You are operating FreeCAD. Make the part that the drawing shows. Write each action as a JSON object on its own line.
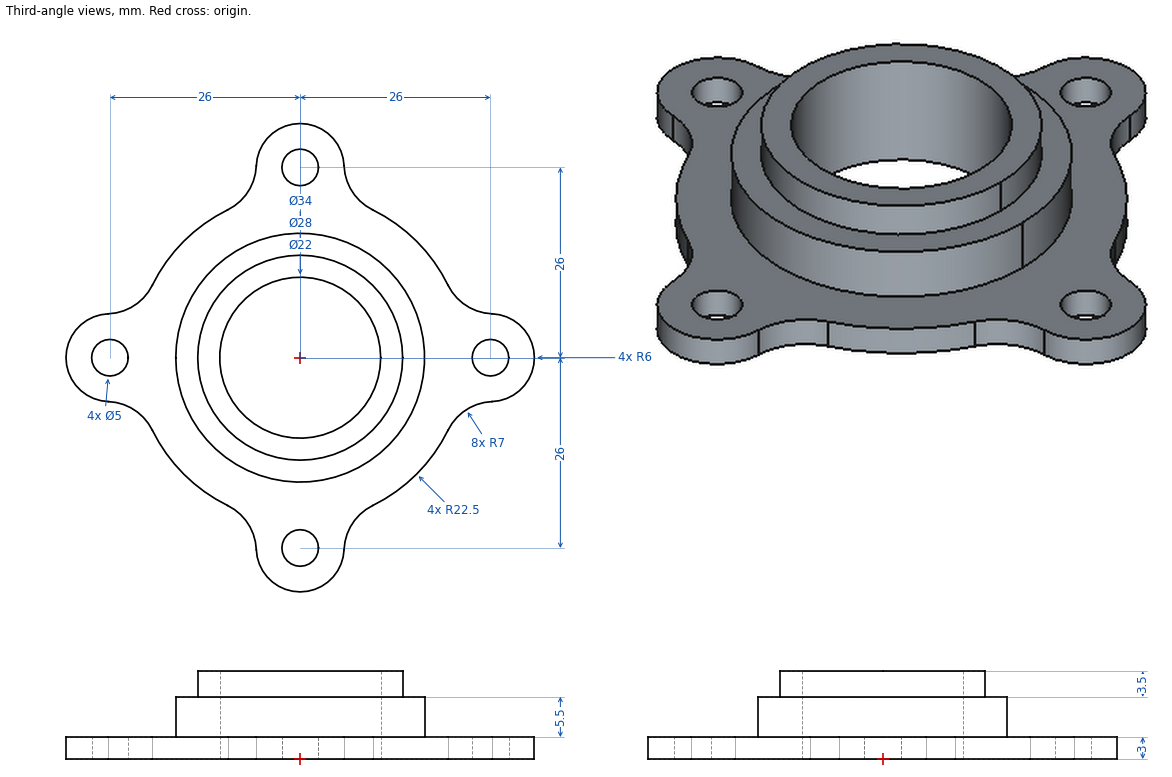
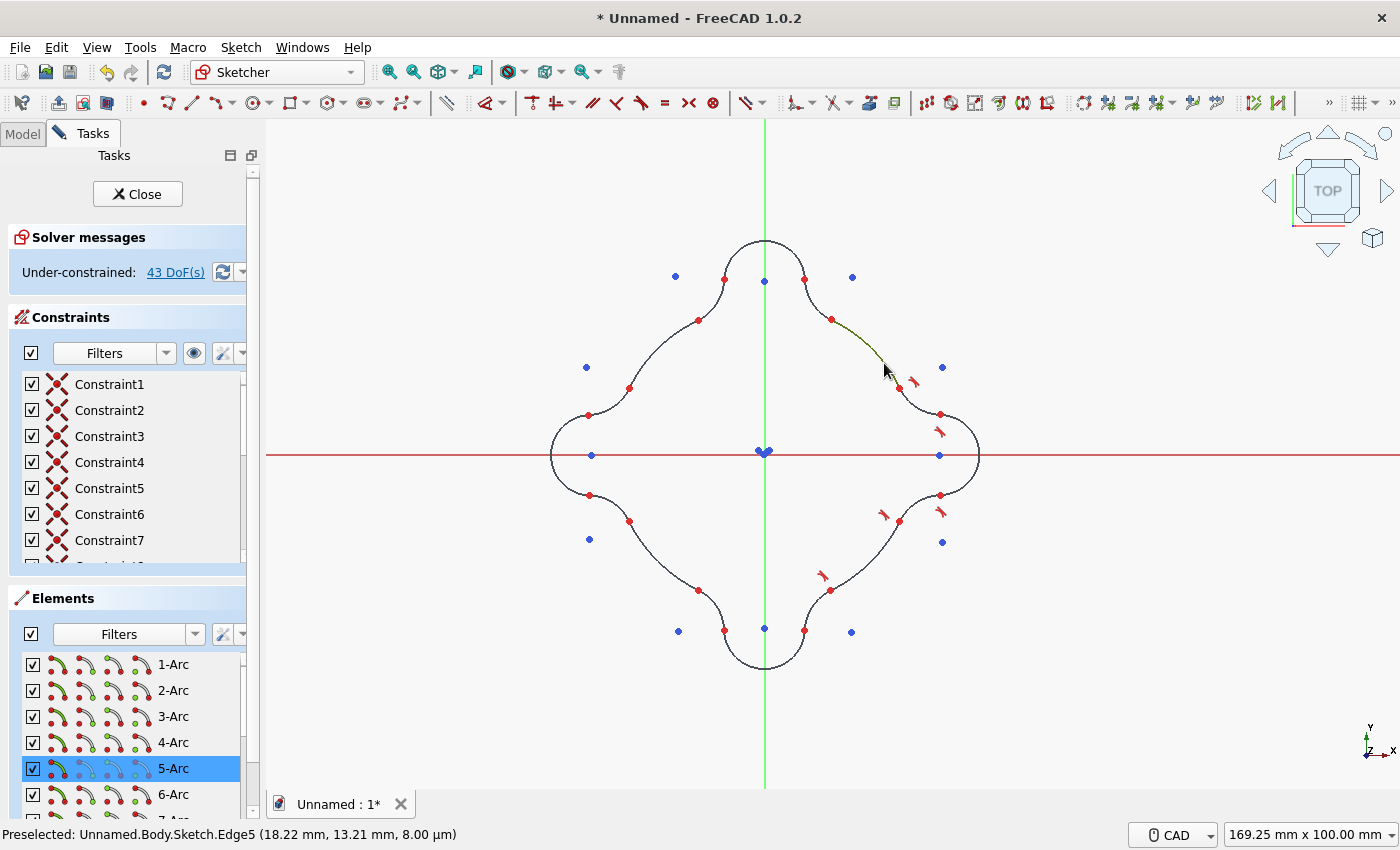
{"action": "left_click", "coordinate": [808, 294]}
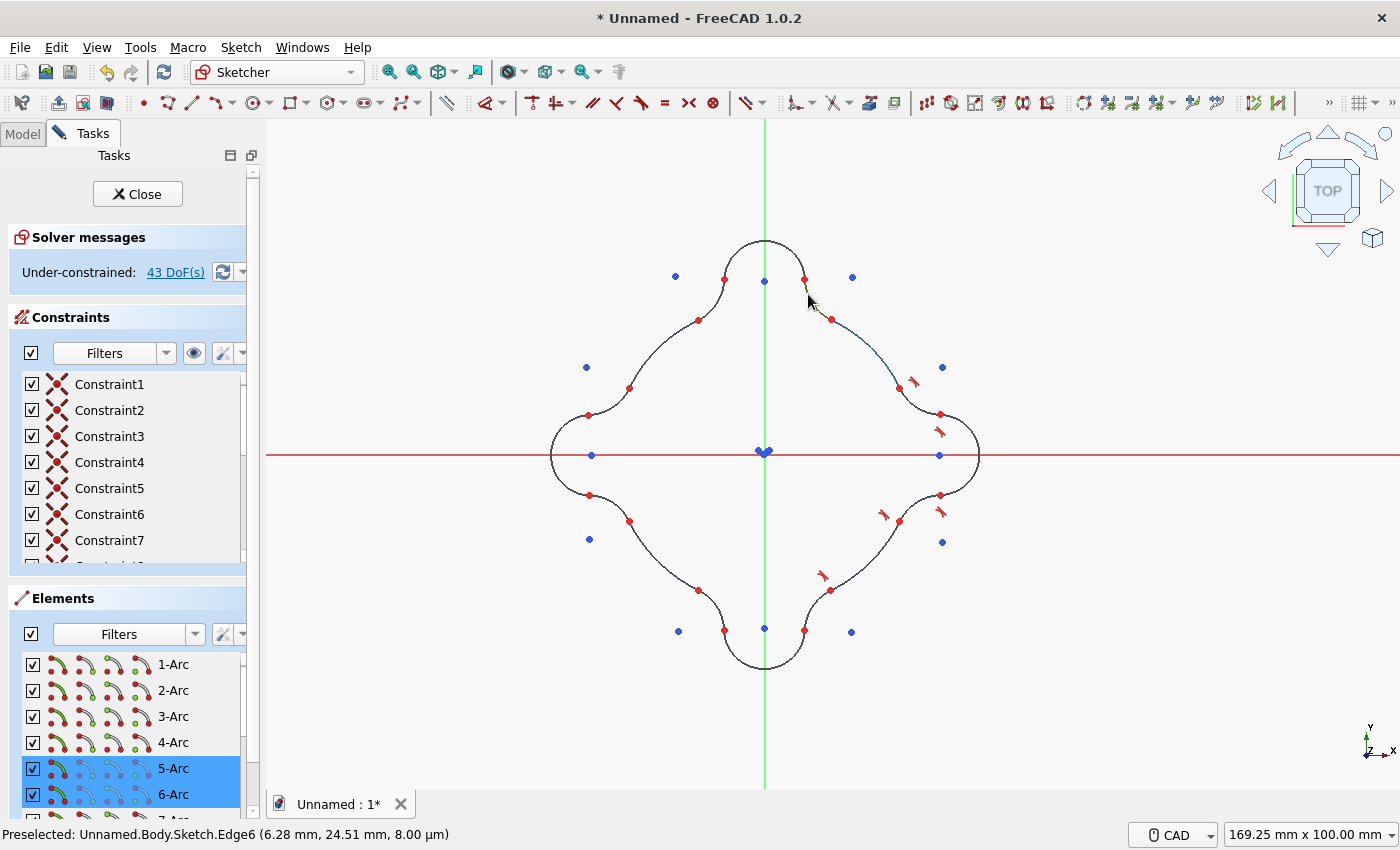
{"action": "left_click", "coordinate": [642, 104]}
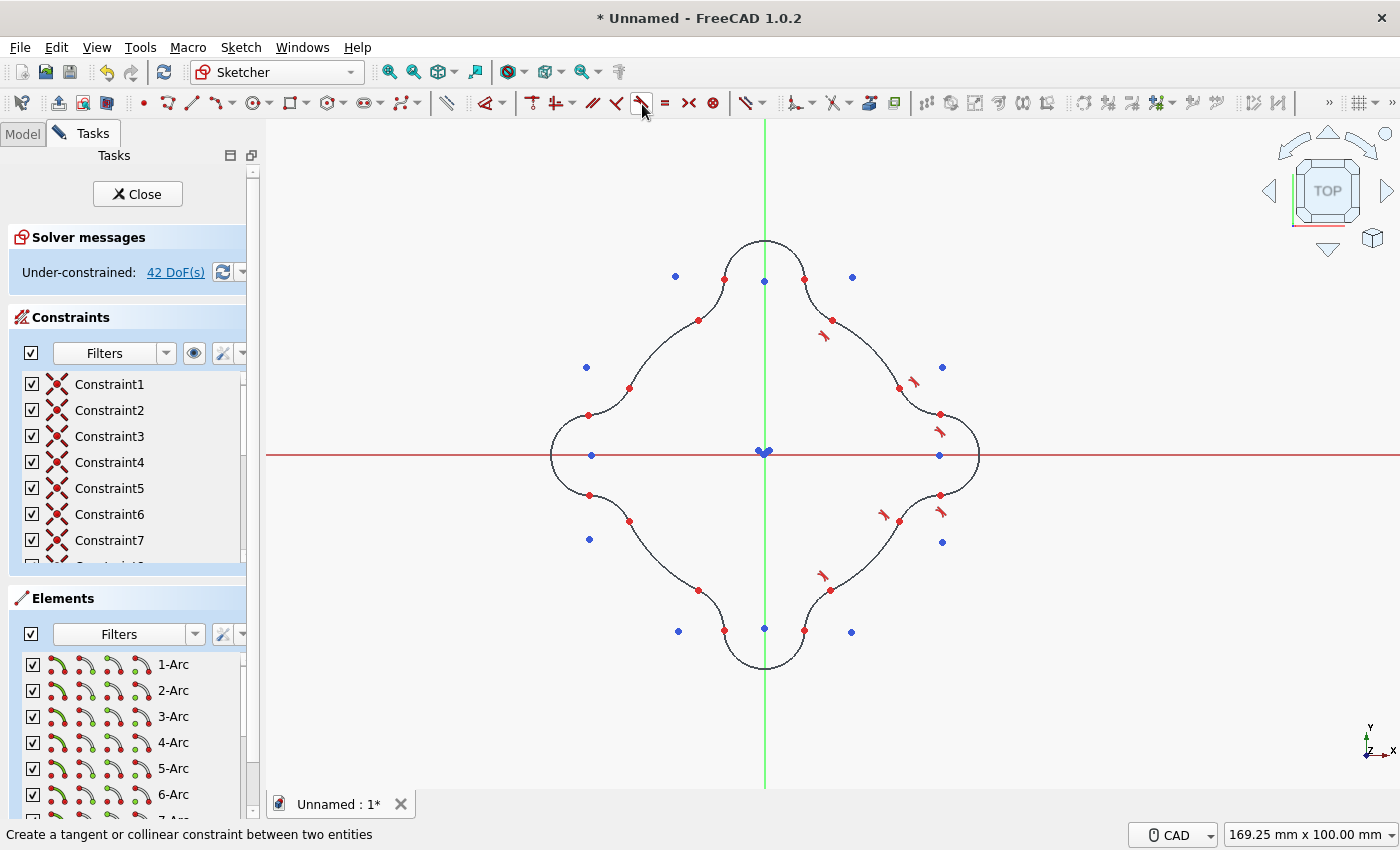
{"action": "left_click", "coordinate": [808, 295]}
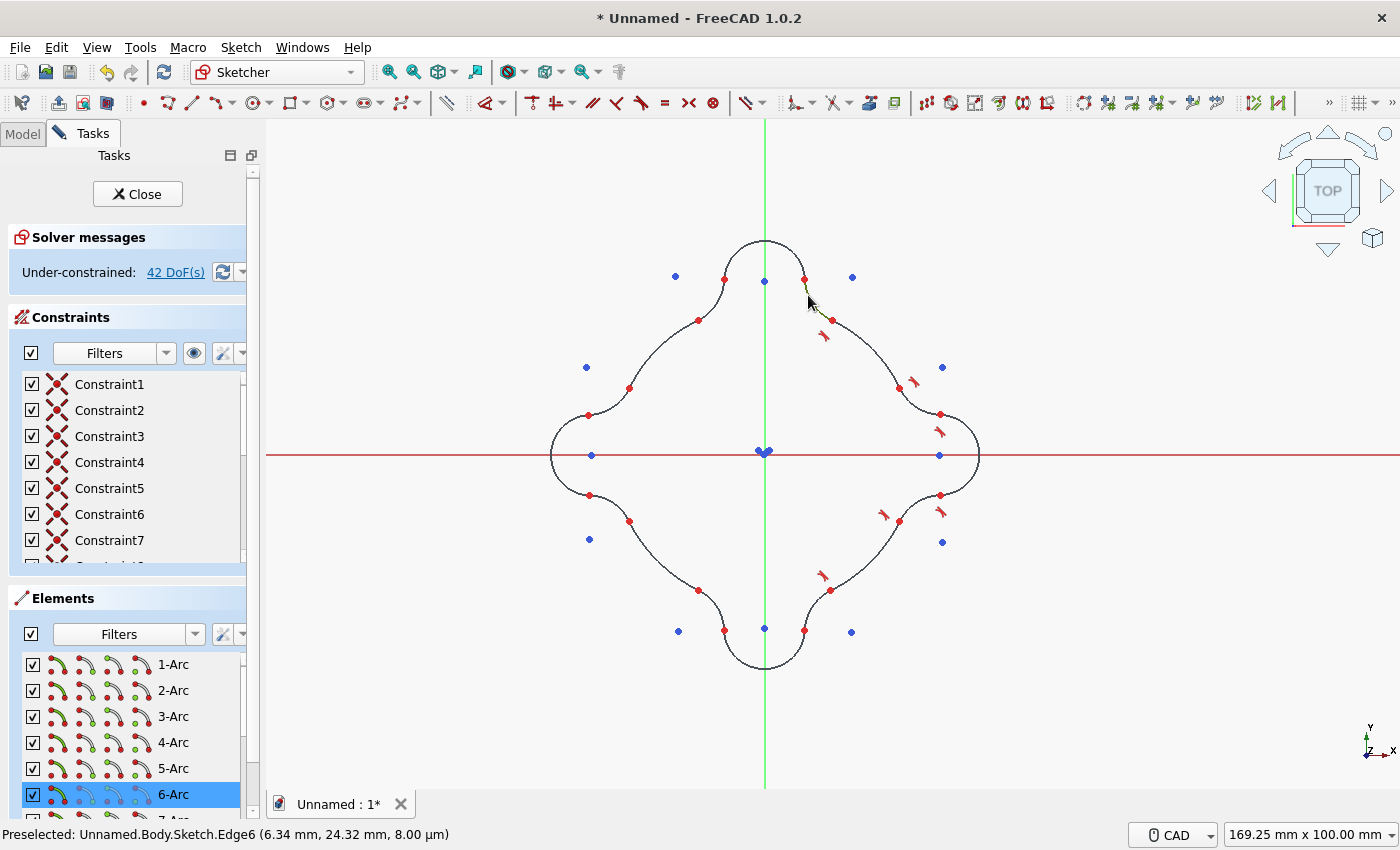
{"action": "left_click", "coordinate": [788, 248]}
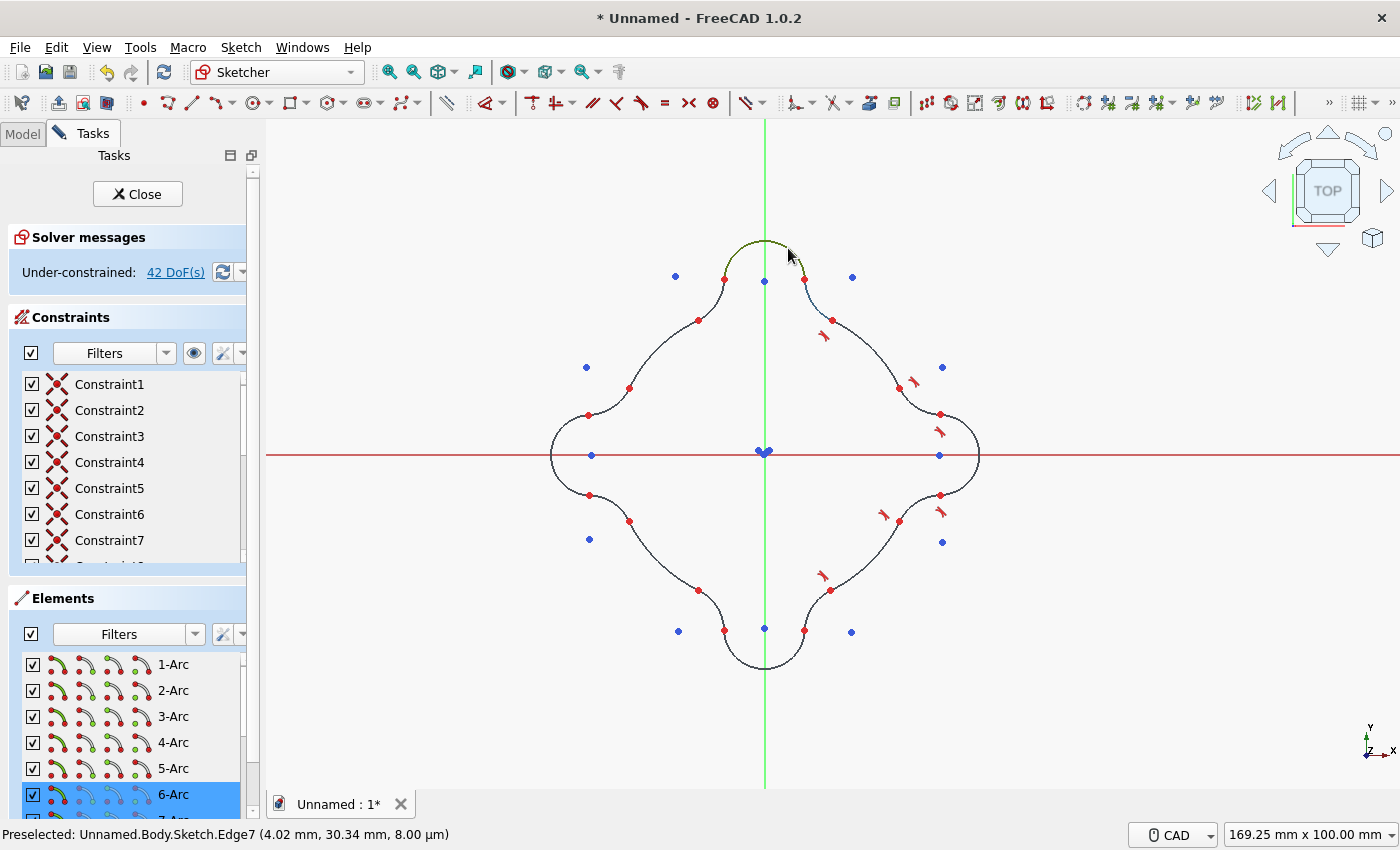
{"action": "left_click", "coordinate": [642, 104]}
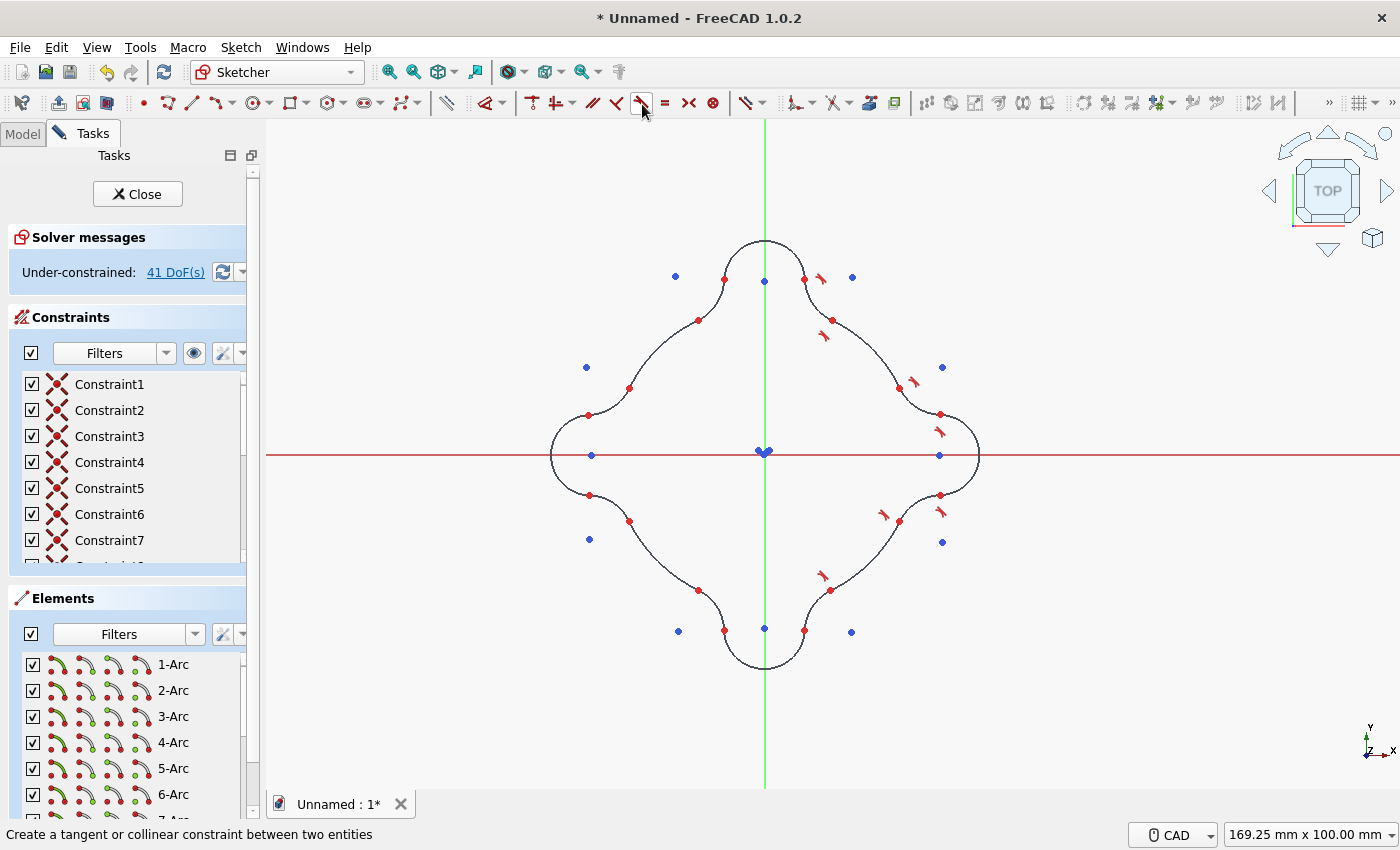
{"action": "left_click", "coordinate": [788, 248]}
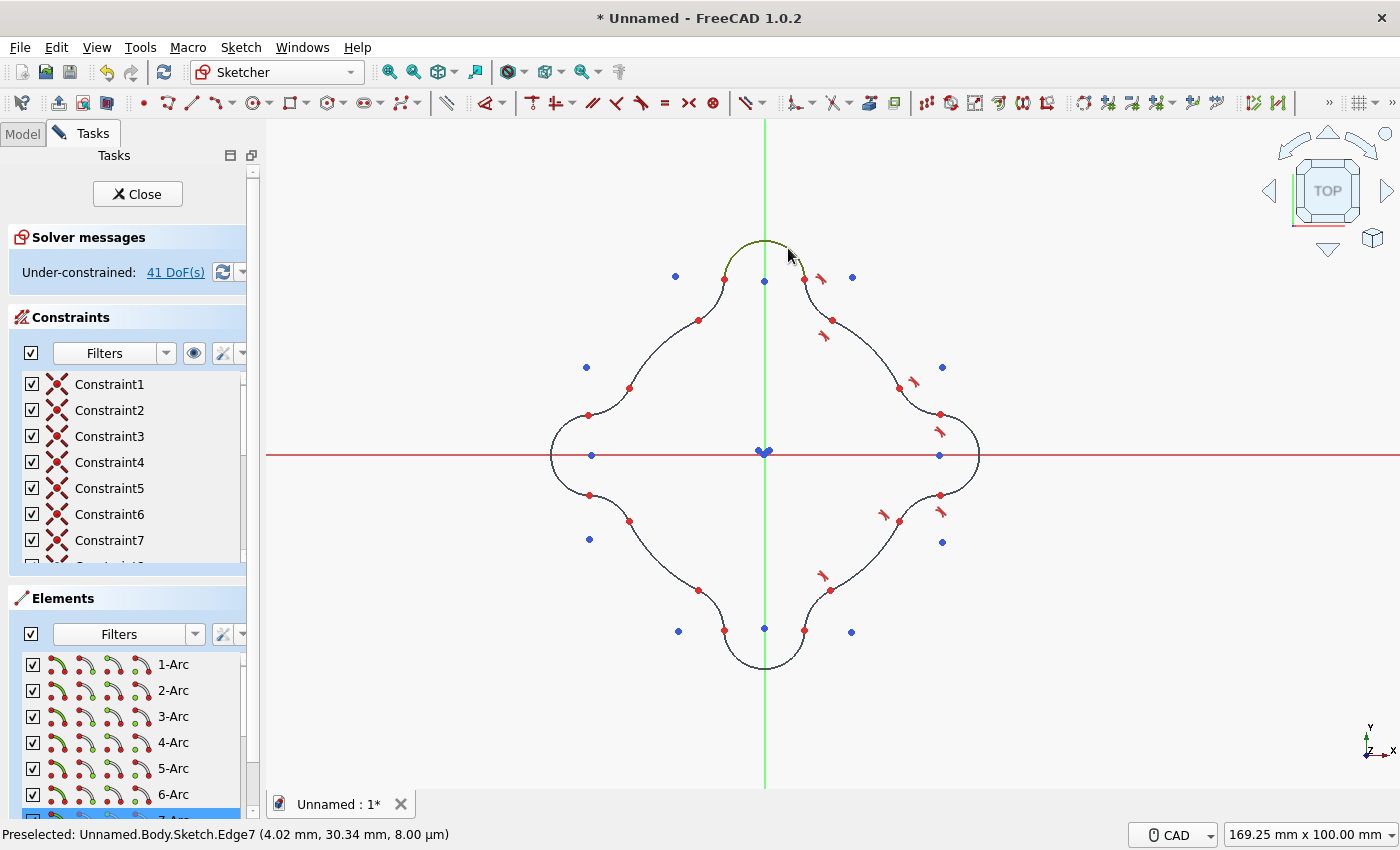
{"action": "left_click", "coordinate": [710, 312]}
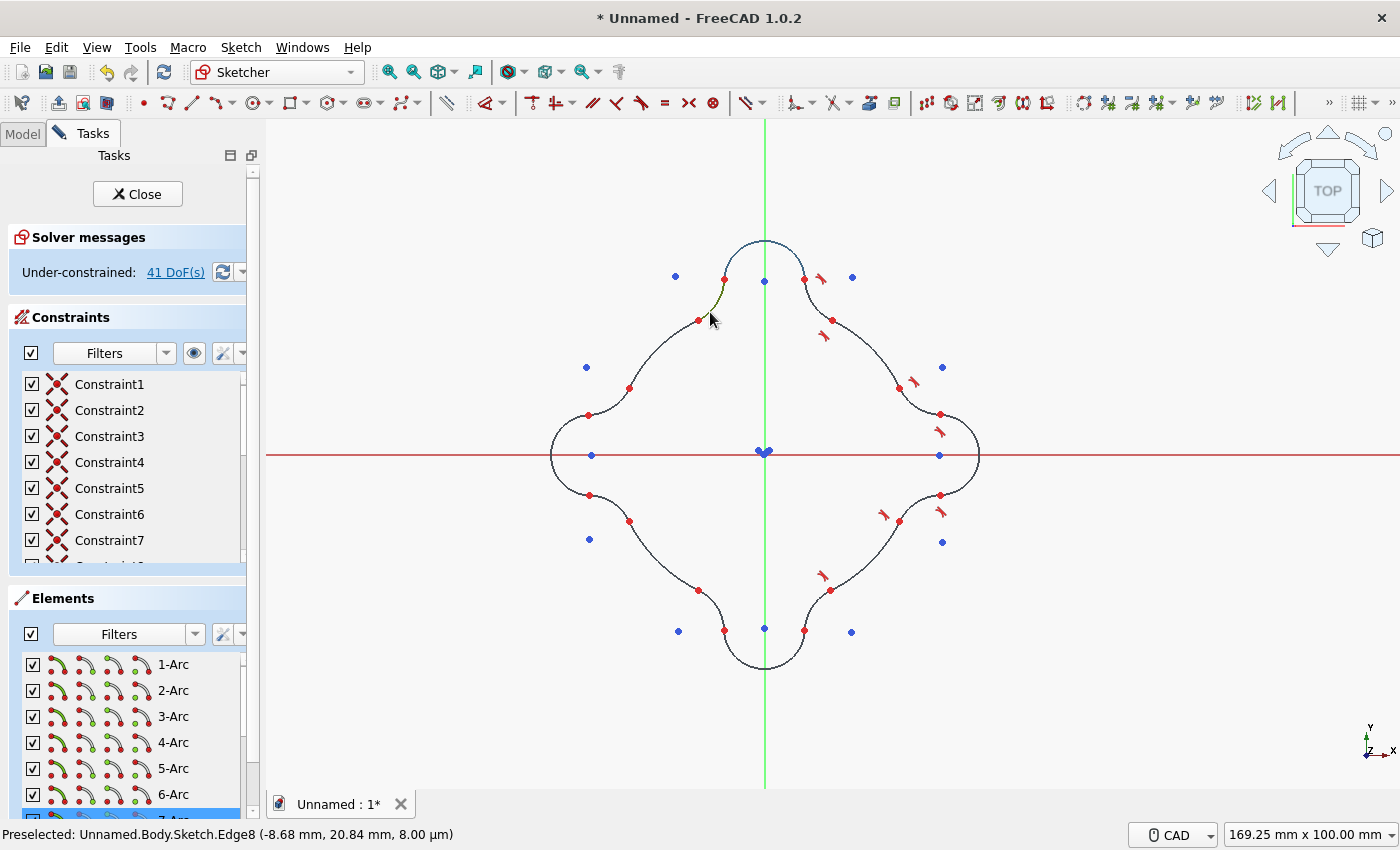
{"action": "left_click", "coordinate": [642, 104]}